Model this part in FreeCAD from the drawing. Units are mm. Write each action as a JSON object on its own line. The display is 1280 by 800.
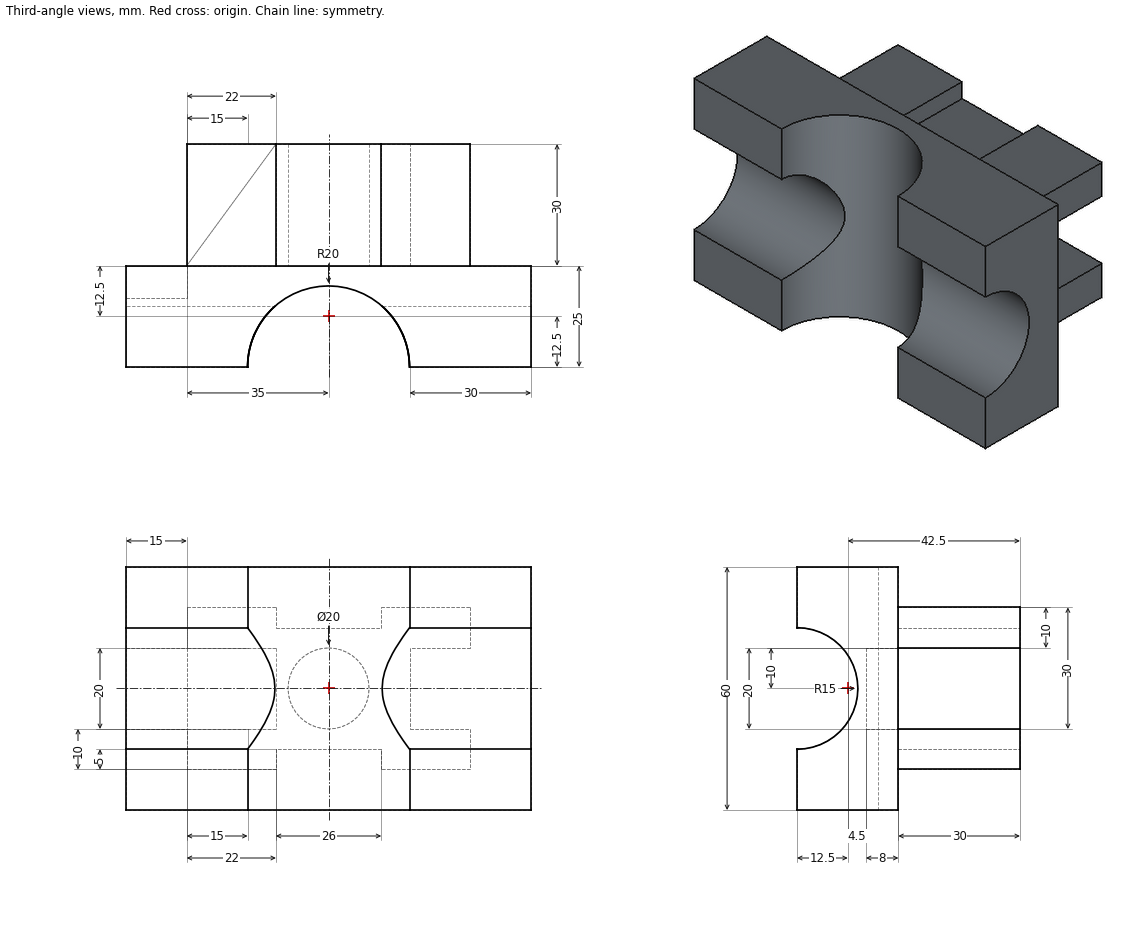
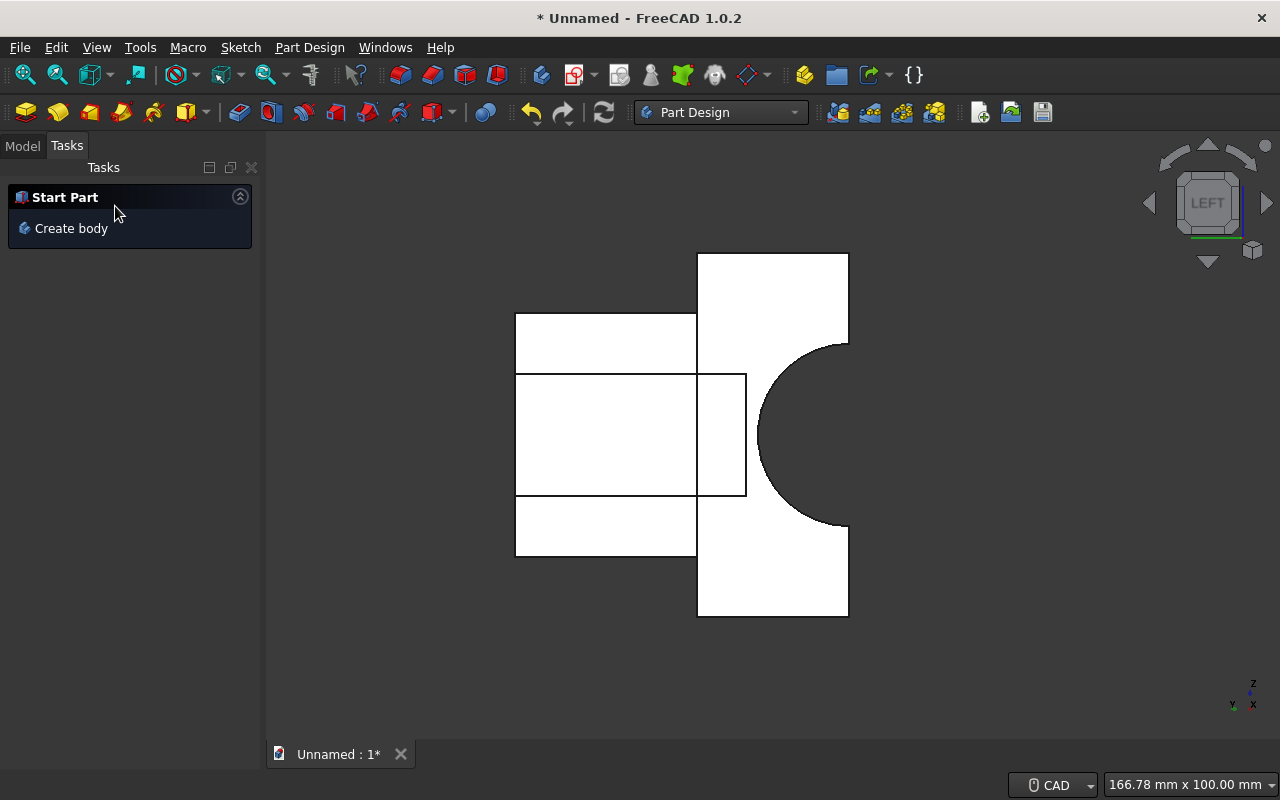
{"action": "left_click", "coordinate": [580, 434]}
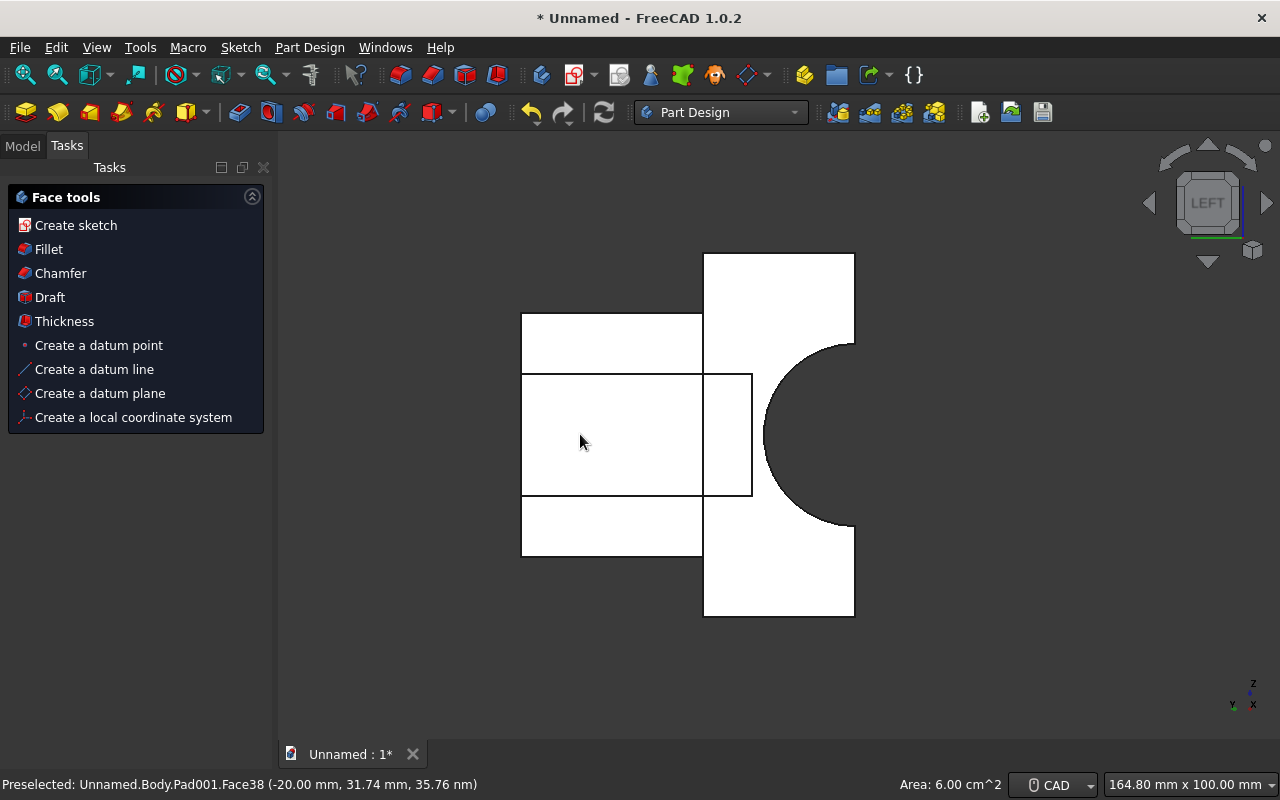
{"action": "left_click", "coordinate": [574, 76]}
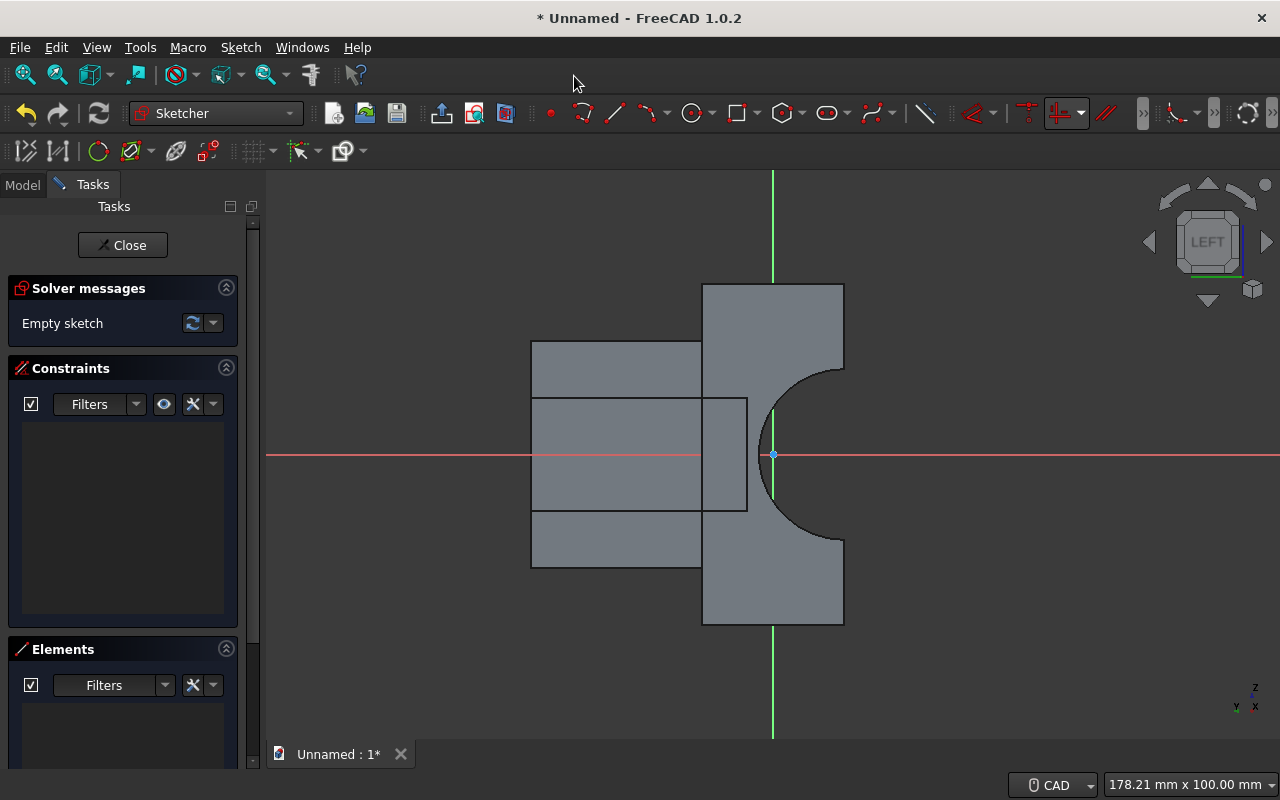
{"action": "scroll", "coordinate": [609, 455], "scroll_direction": "up", "scroll_amount": 4}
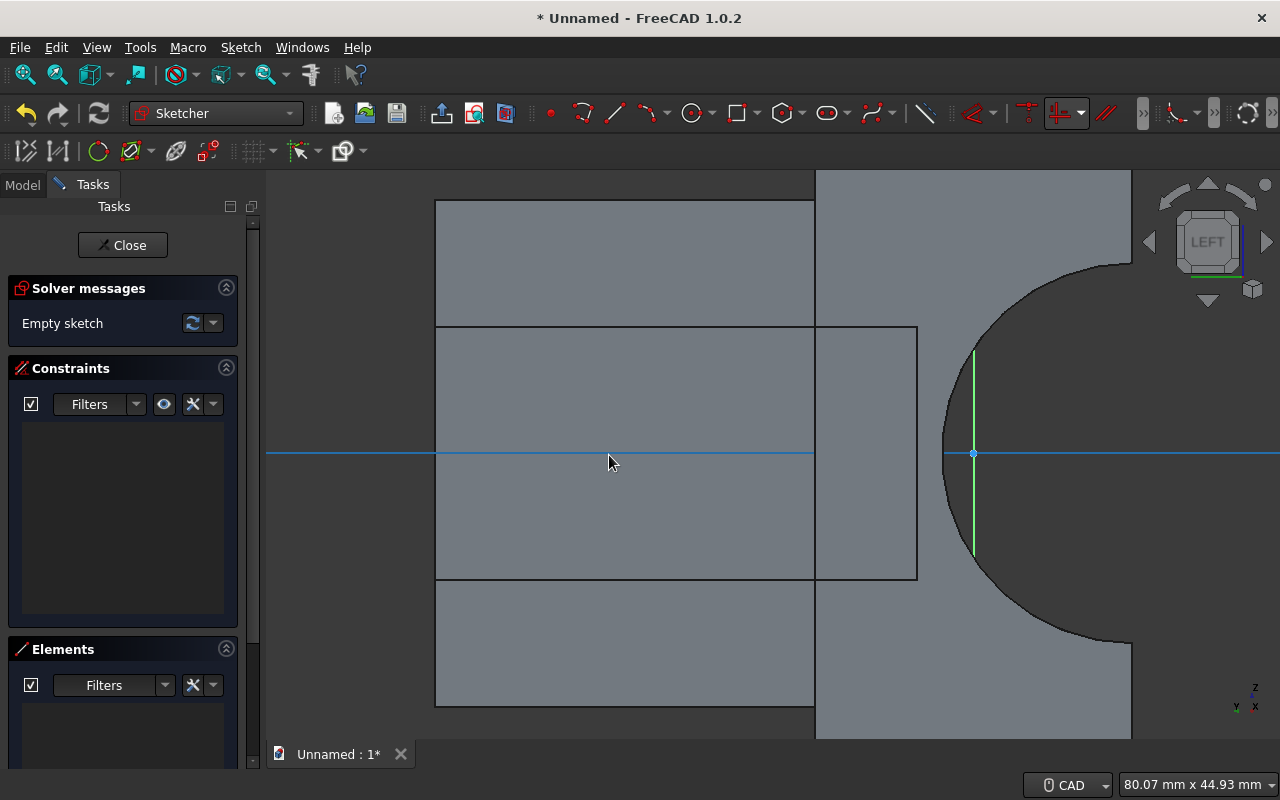
{"action": "left_click", "coordinate": [738, 114]}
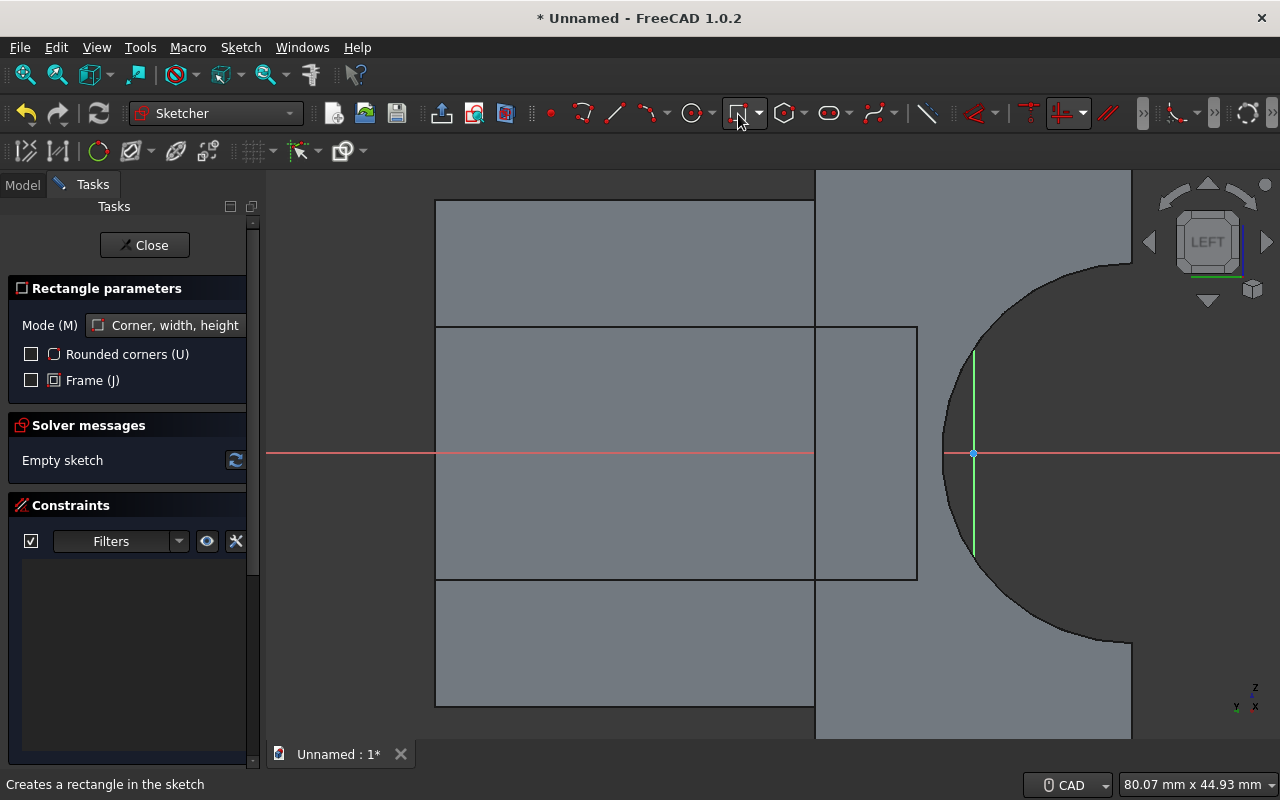
{"action": "left_click", "coordinate": [435, 327]}
{"action": "left_click", "coordinate": [815, 580]}
{"action": "key", "text": "Escape"}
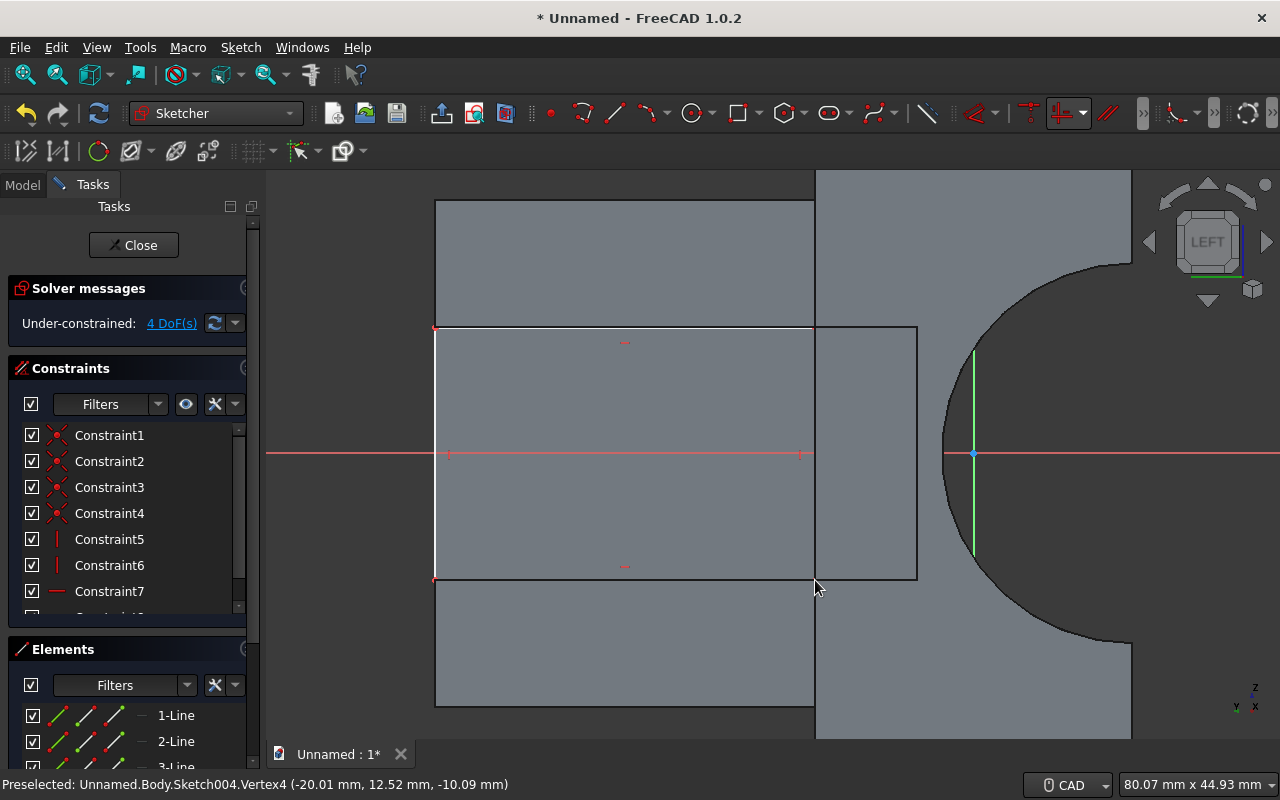
{"action": "key", "text": "d"}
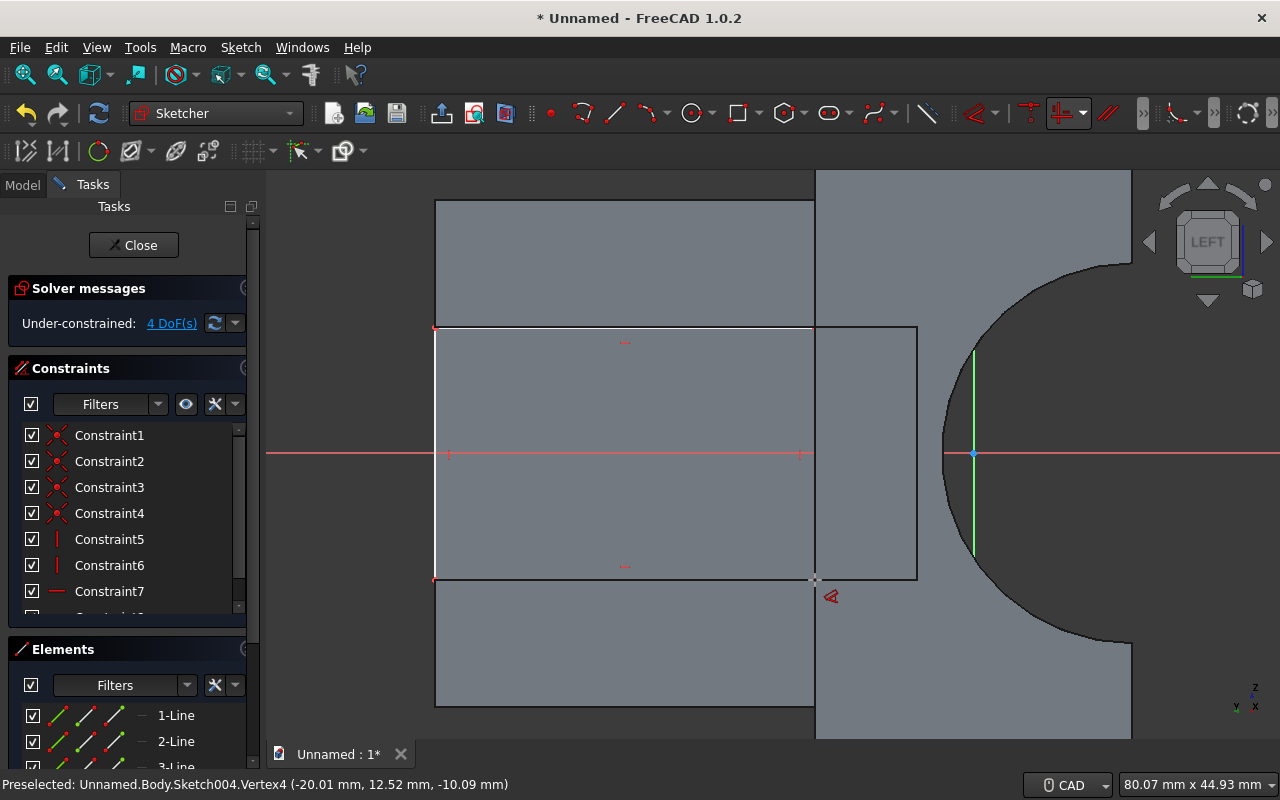
{"action": "left_click", "coordinate": [435, 404]}
{"action": "left_click", "coordinate": [401, 396]}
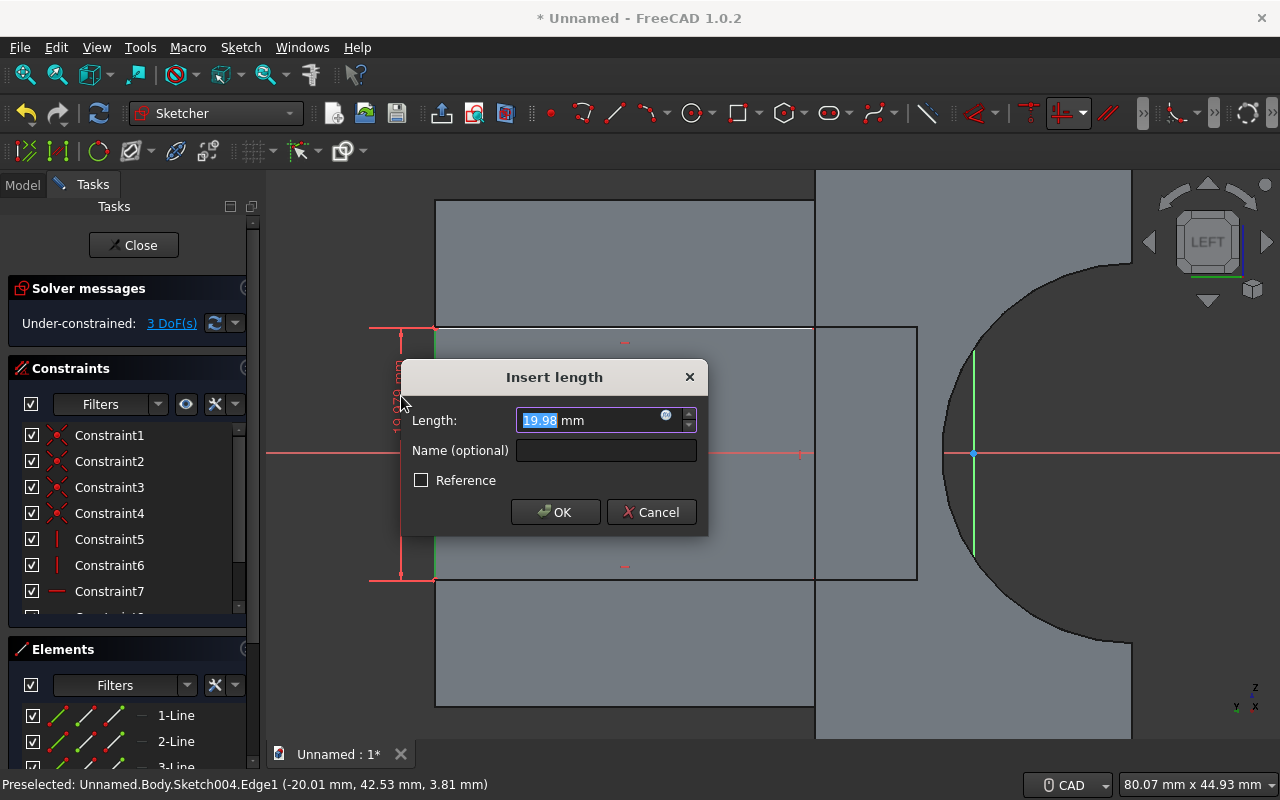
{"action": "type", "text": "20"}
{"action": "key", "text": "Return"}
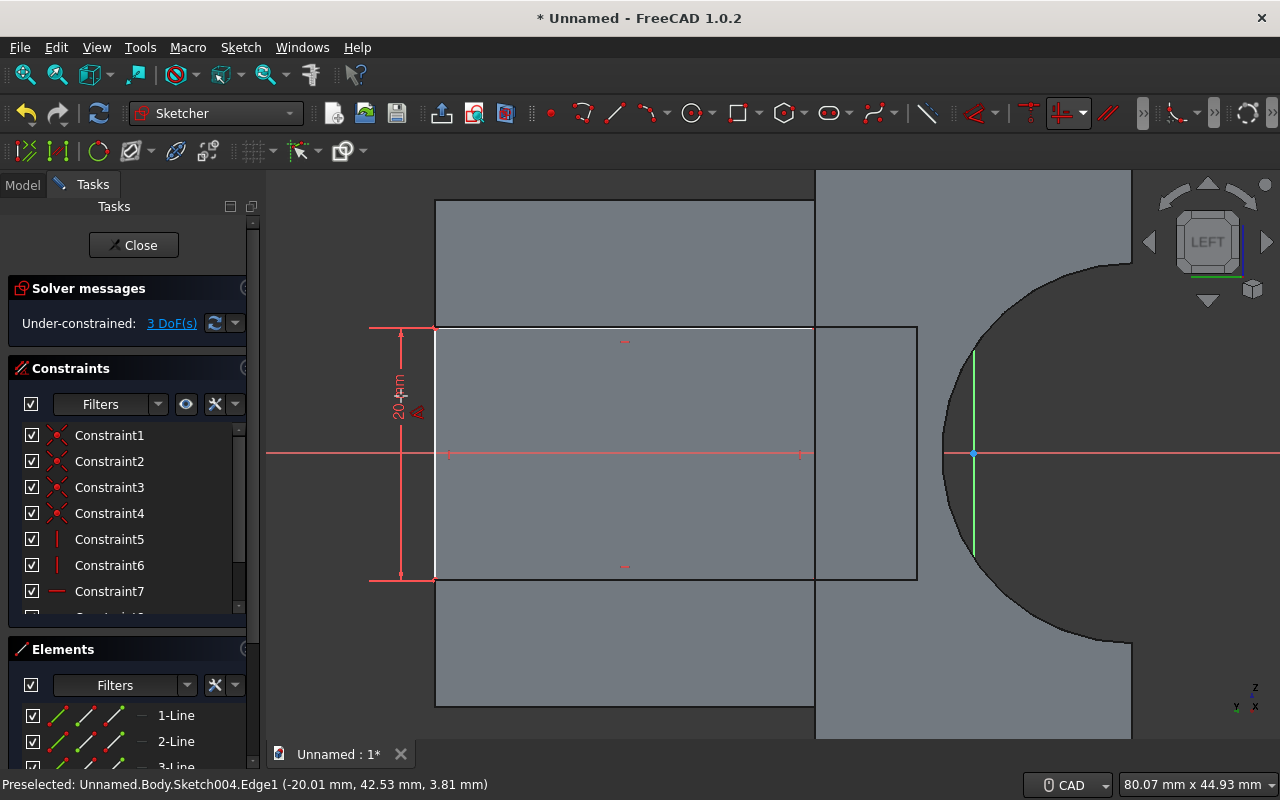
{"action": "left_click", "coordinate": [549, 581]}
{"action": "left_click", "coordinate": [625, 615]}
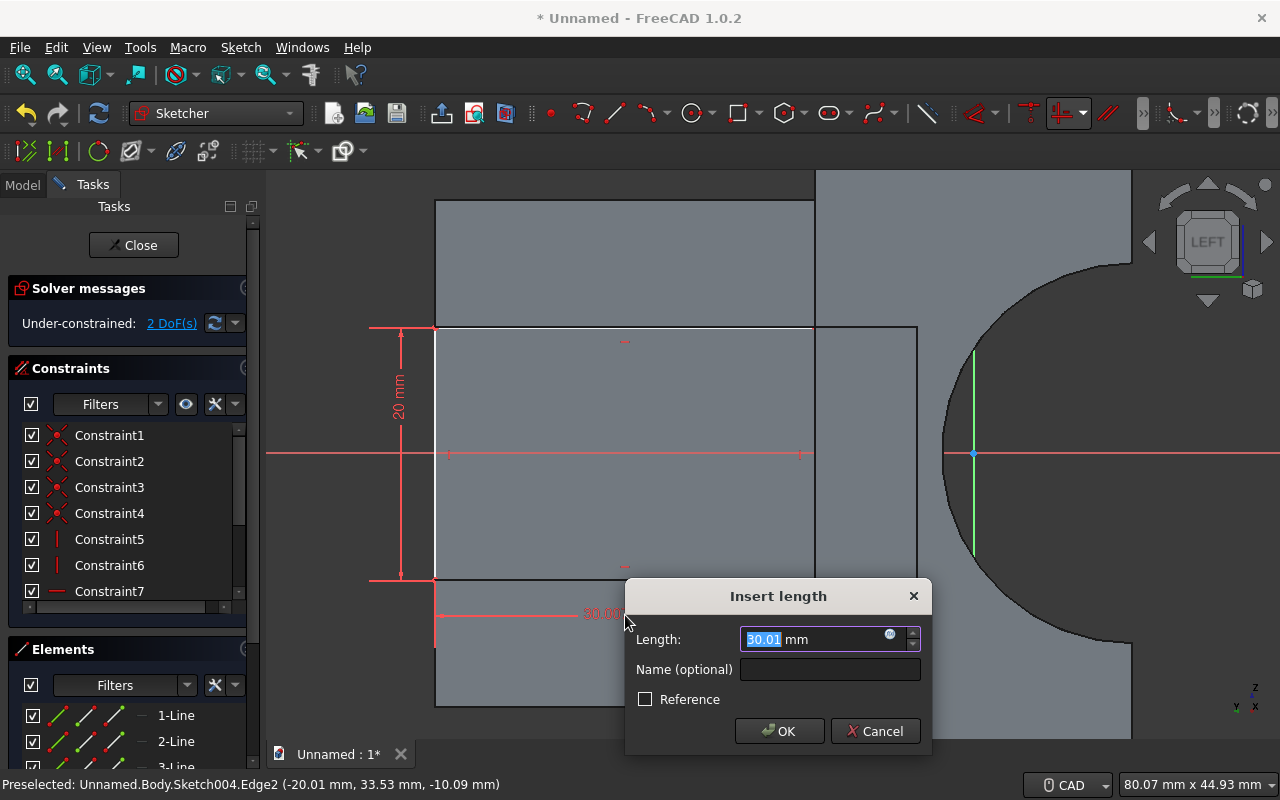
{"action": "type", "text": "30"}
{"action": "key", "text": "Return"}